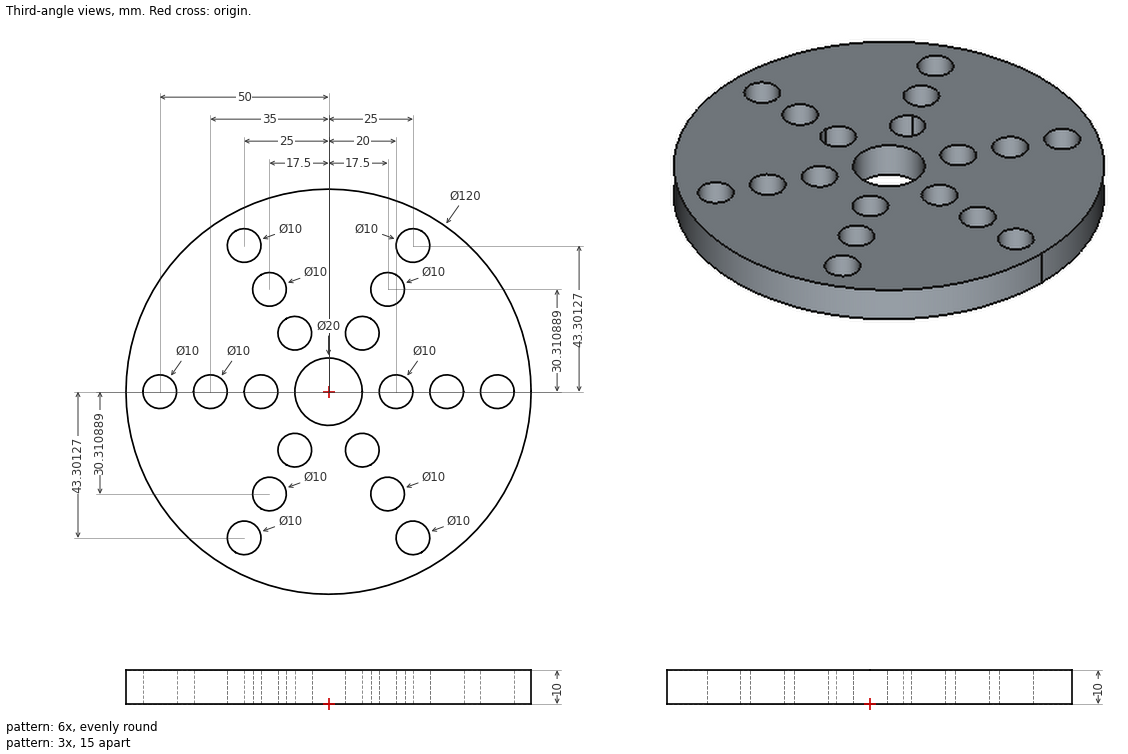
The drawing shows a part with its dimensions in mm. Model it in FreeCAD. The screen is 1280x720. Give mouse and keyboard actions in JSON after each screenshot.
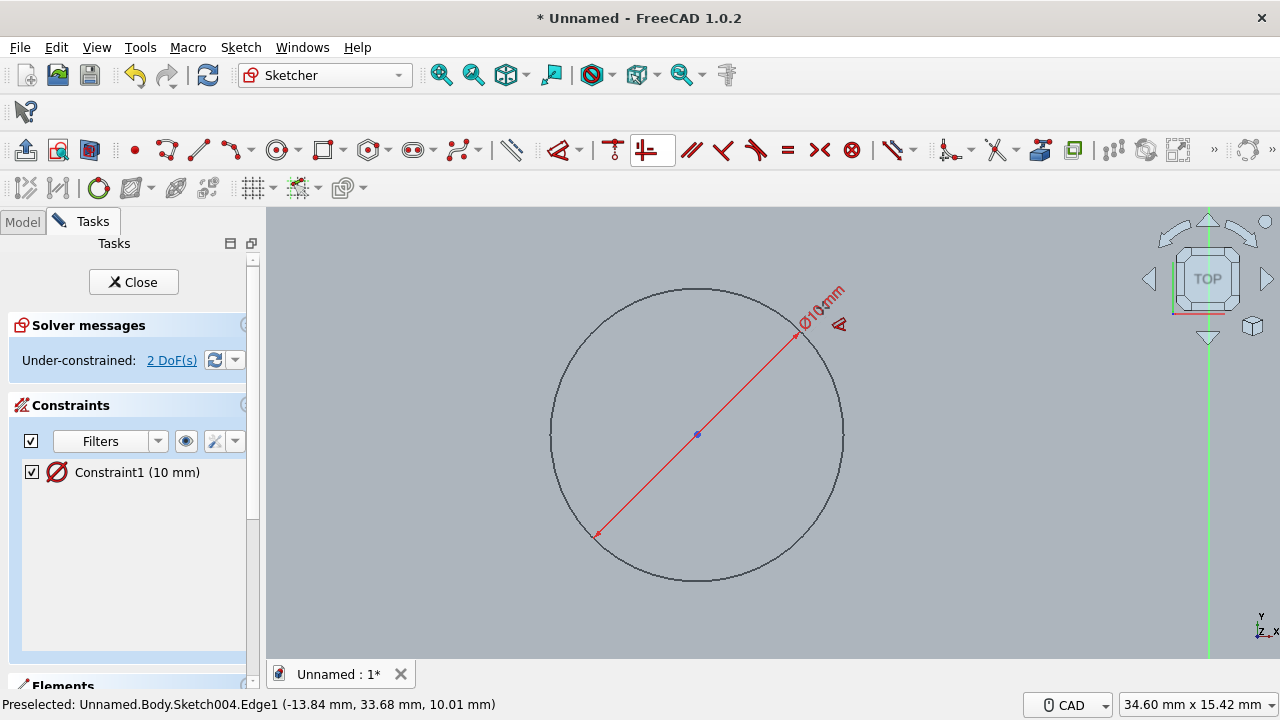
{"action": "left_click", "coordinate": [697, 435]}
{"action": "left_click", "coordinate": [906, 401]}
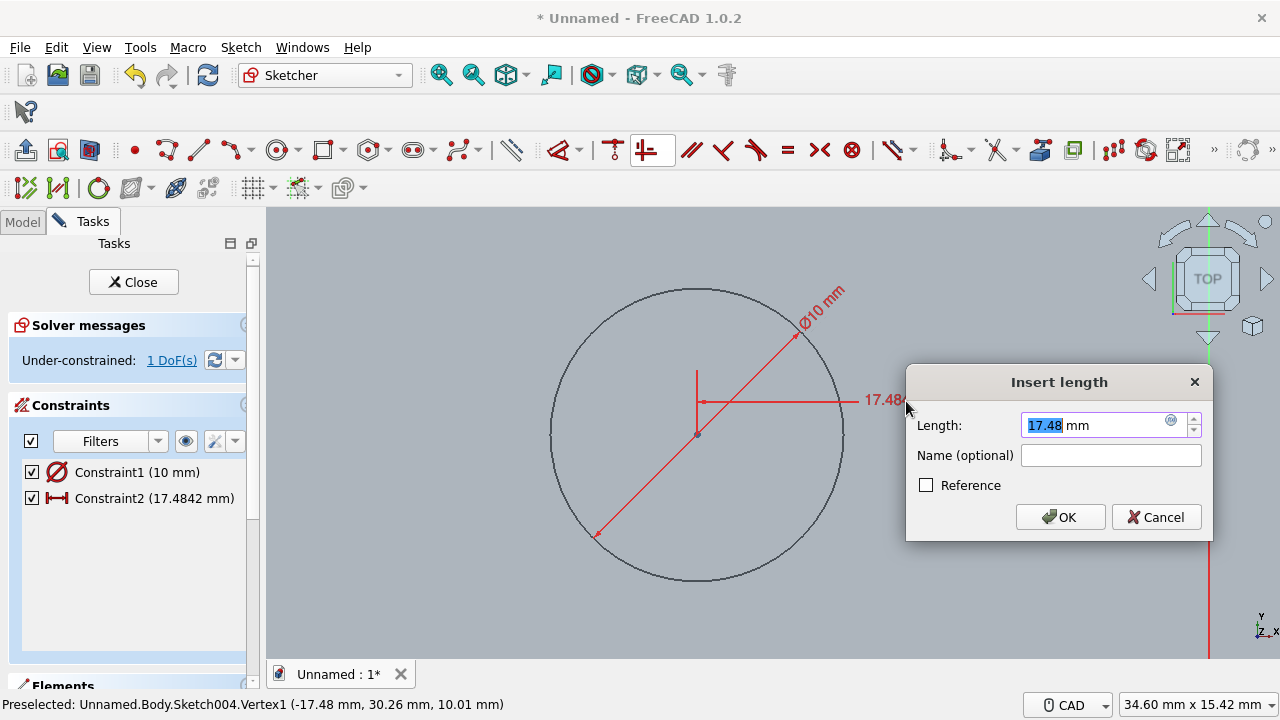
{"action": "type", "text": "17.5"}
{"action": "key", "text": "Return"}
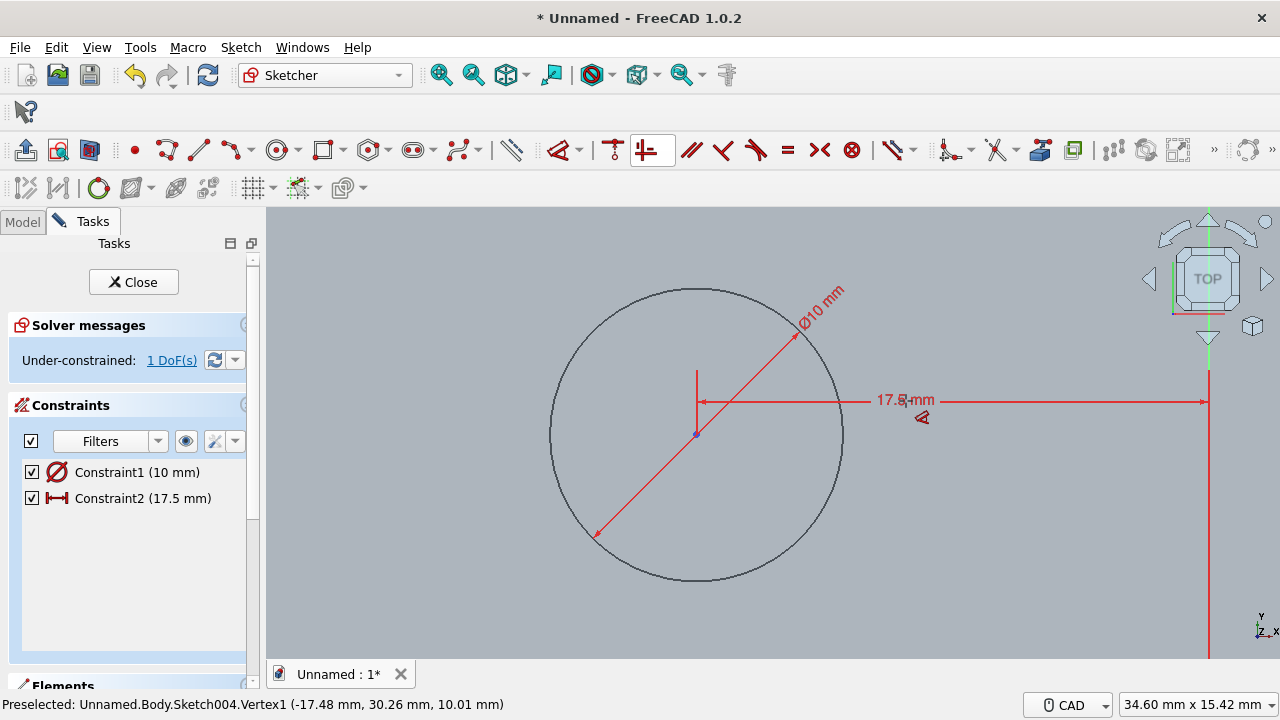
{"action": "left_click", "coordinate": [697, 435]}
{"action": "left_click", "coordinate": [663, 533]}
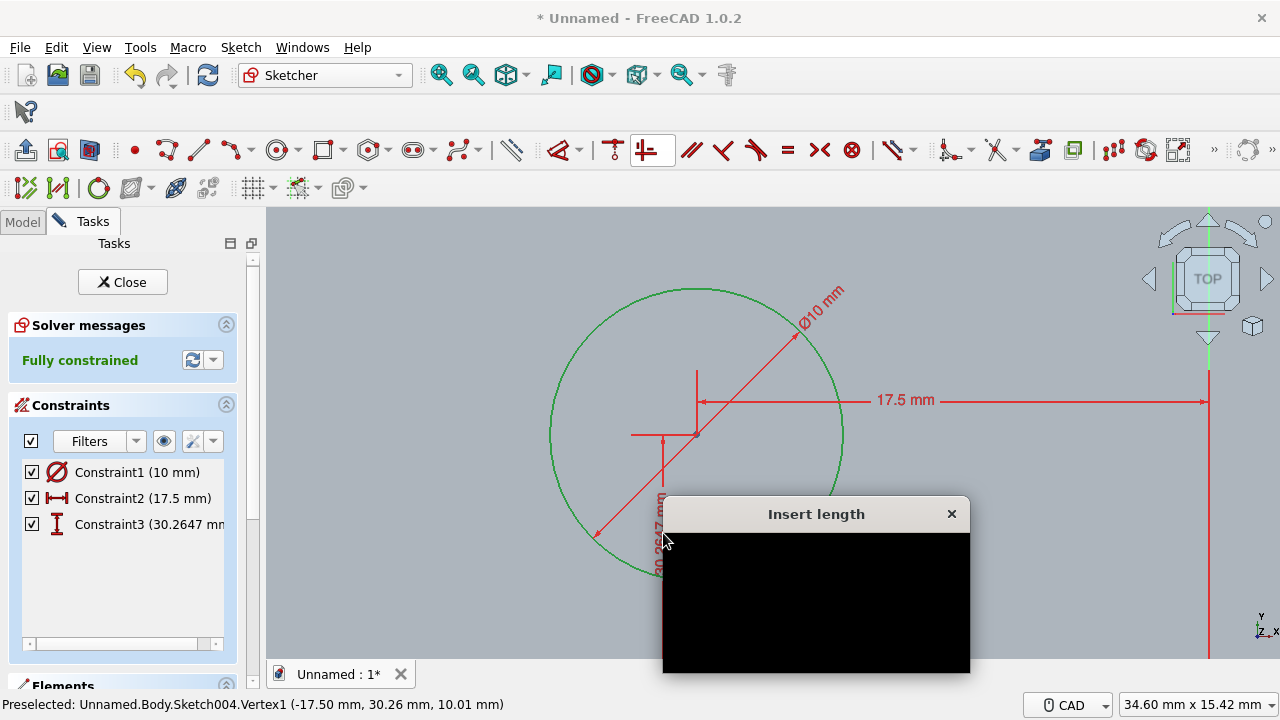
{"action": "type", "text": "30.310889"}
{"action": "key", "text": "Return"}
{"action": "key", "text": "Escape"}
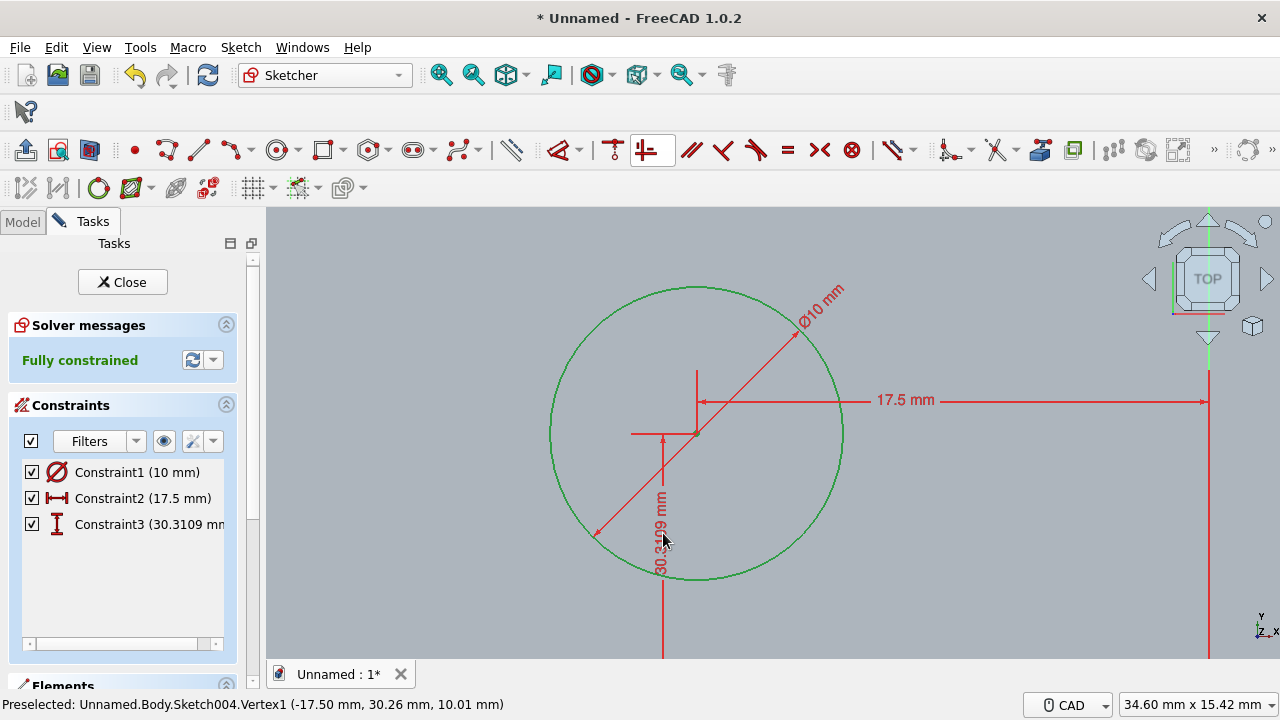
{"action": "left_click", "coordinate": [123, 282]}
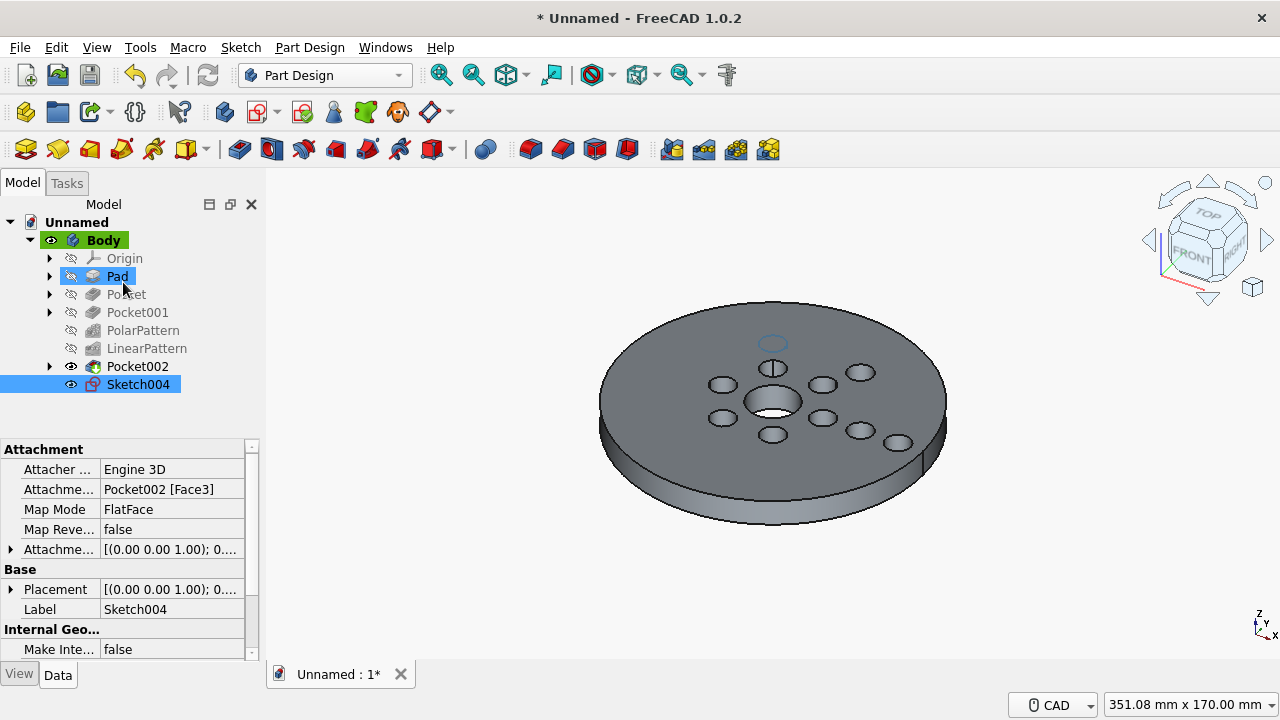
{"action": "left_click", "coordinate": [240, 150]}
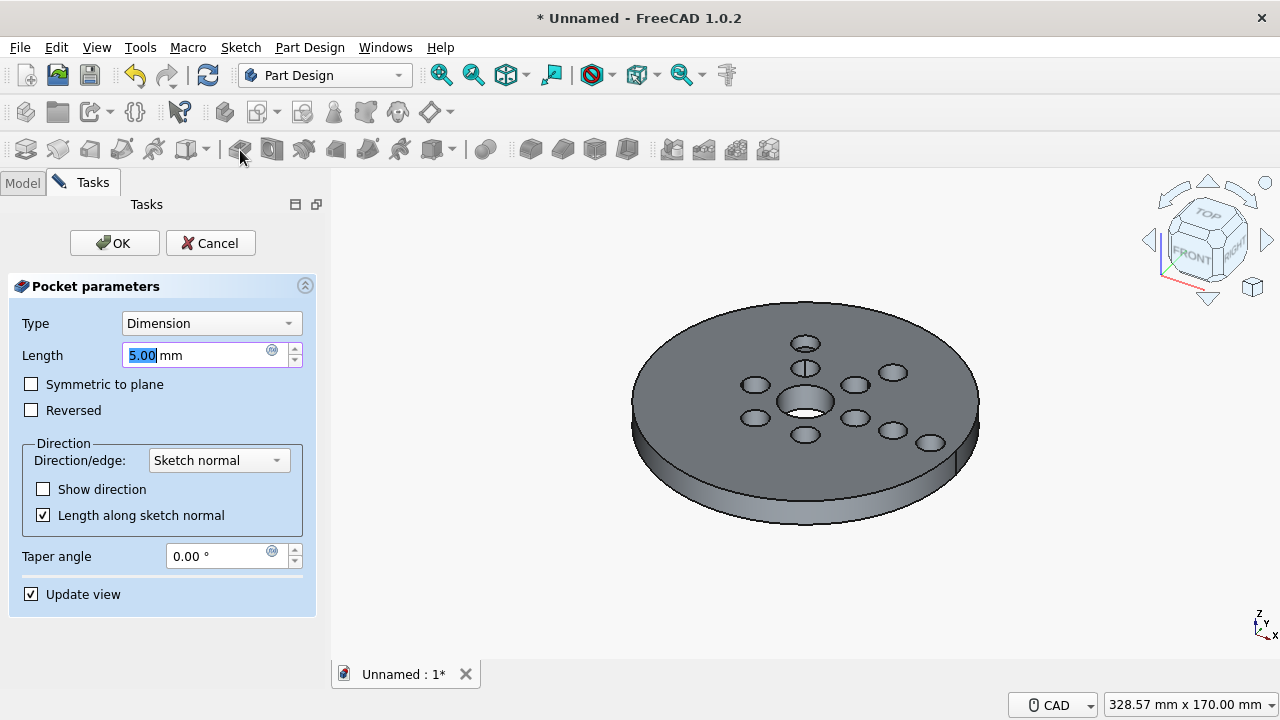
{"action": "type", "text": "10"}
{"action": "key", "text": "Tab"}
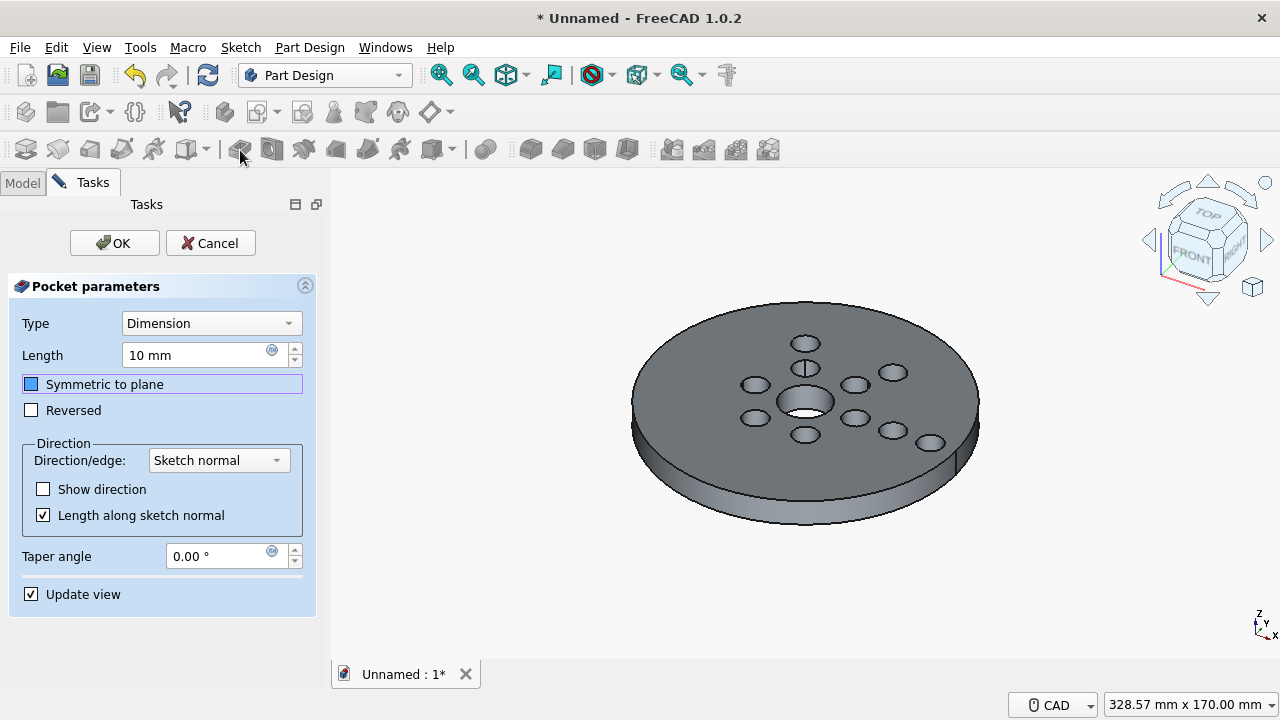
{"action": "left_click", "coordinate": [115, 243]}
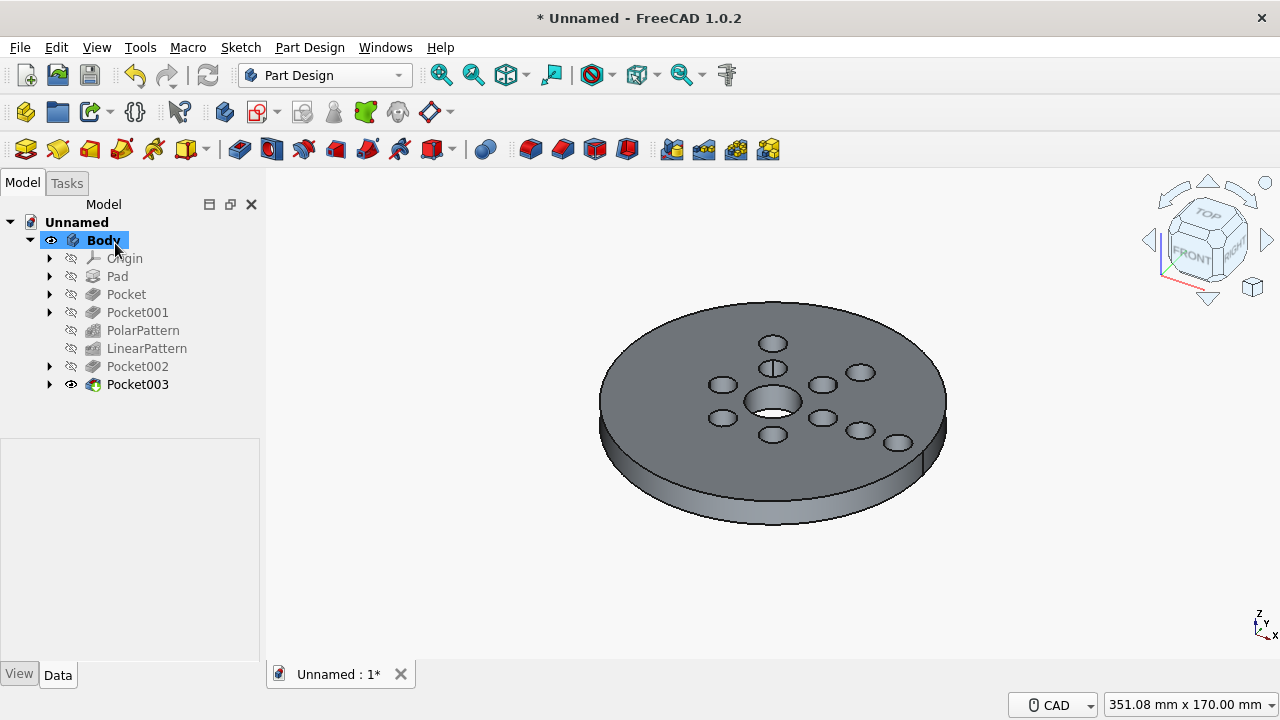
{"action": "left_click", "coordinate": [662, 397]}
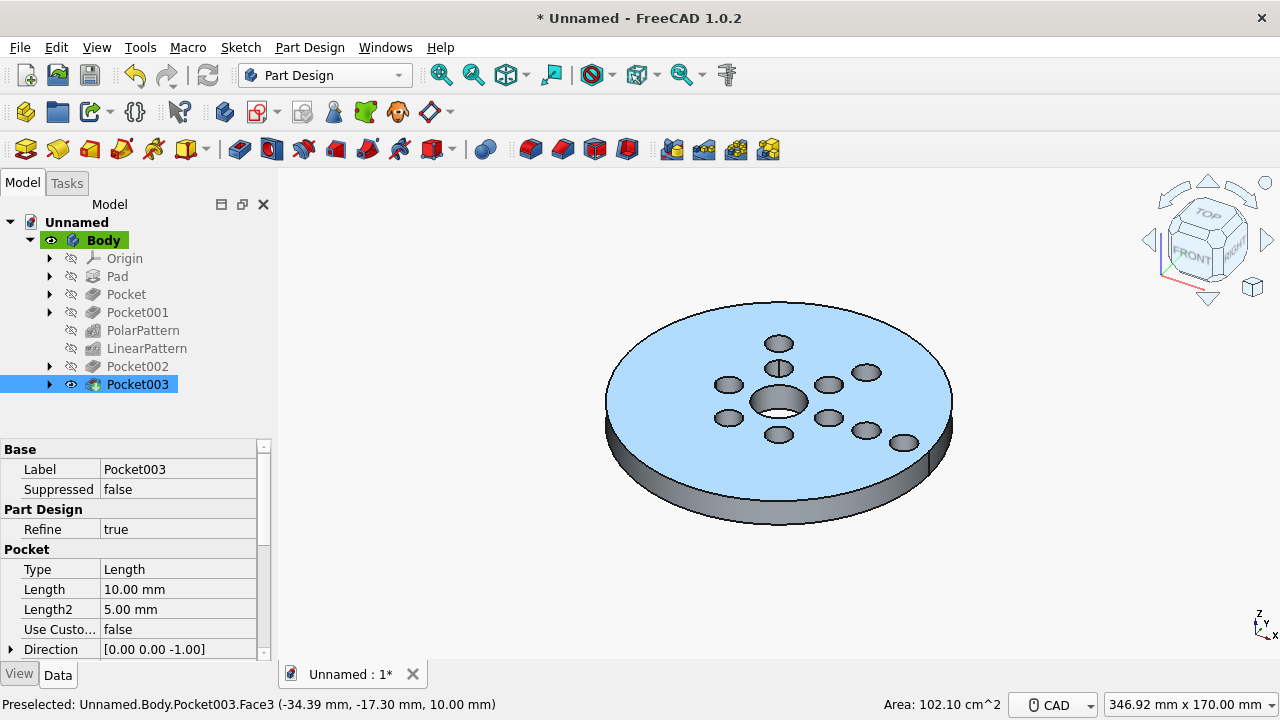
{"action": "left_click", "coordinate": [258, 112]}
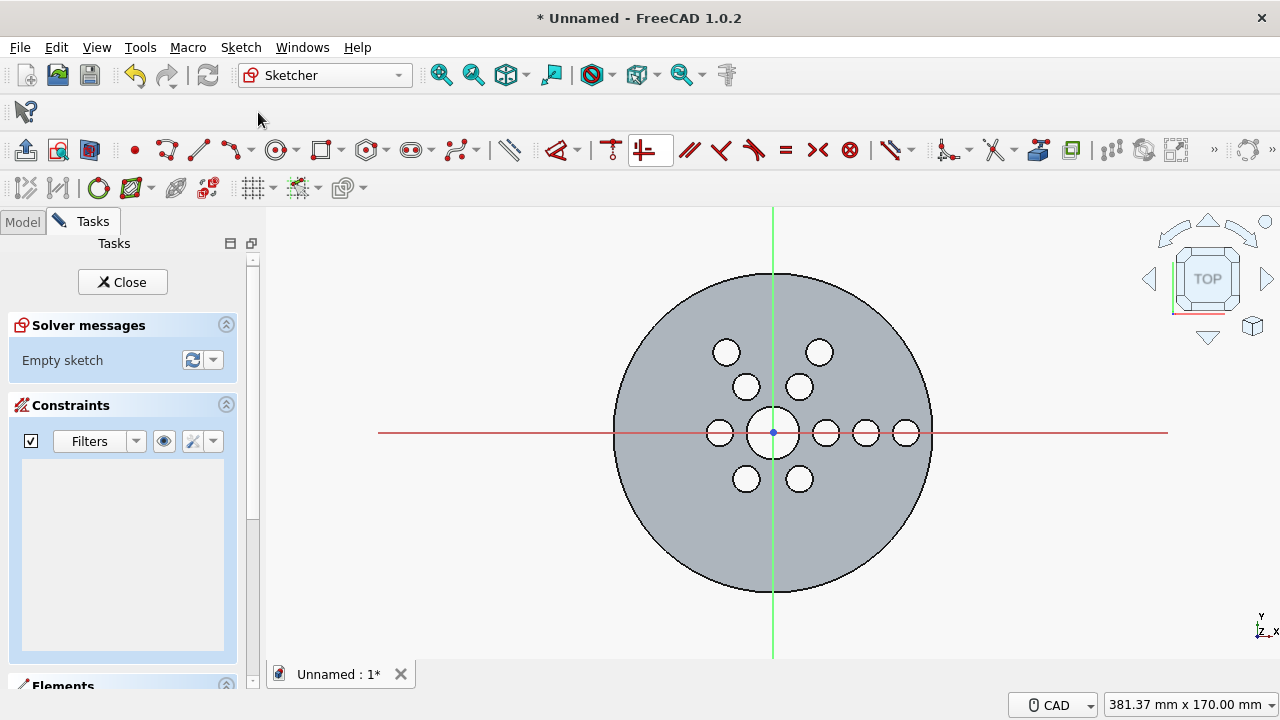
{"action": "scroll", "coordinate": [677, 433], "scroll_direction": "up", "scroll_amount": 12}